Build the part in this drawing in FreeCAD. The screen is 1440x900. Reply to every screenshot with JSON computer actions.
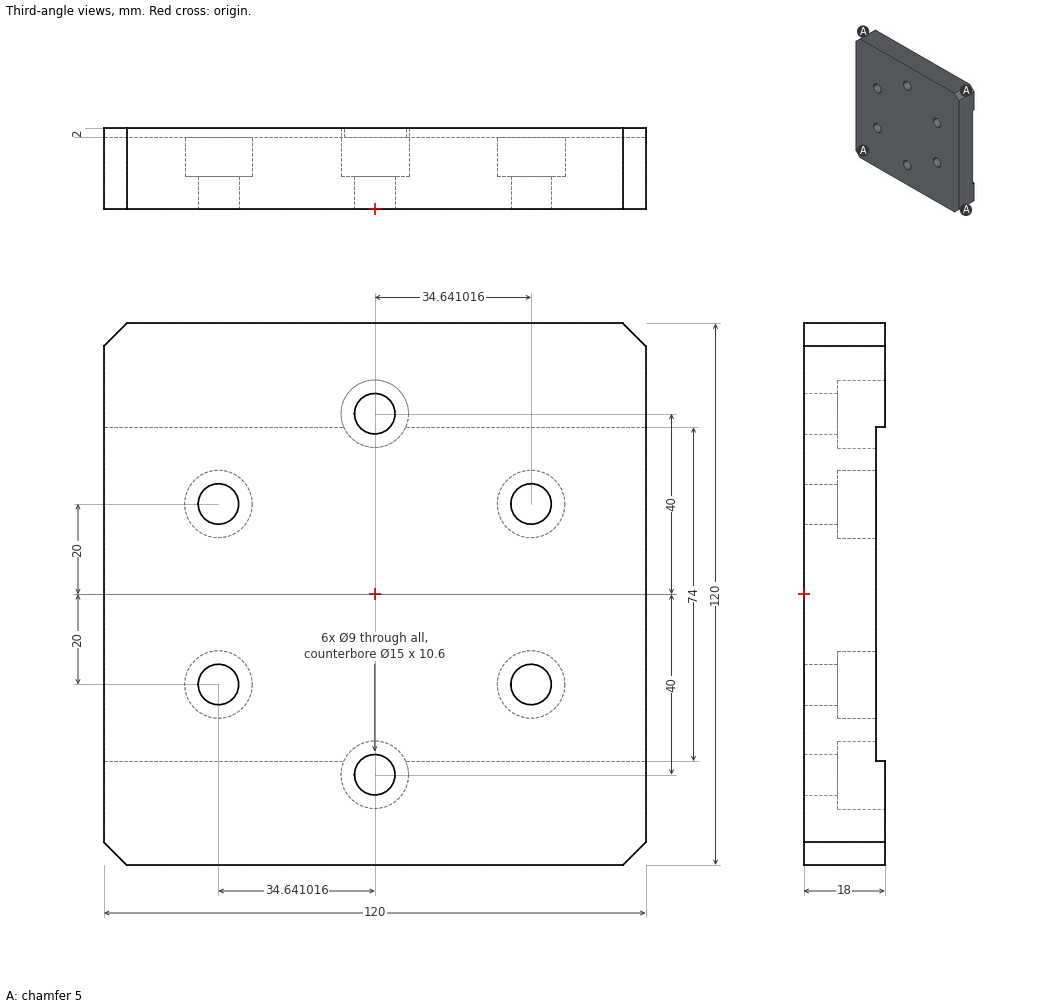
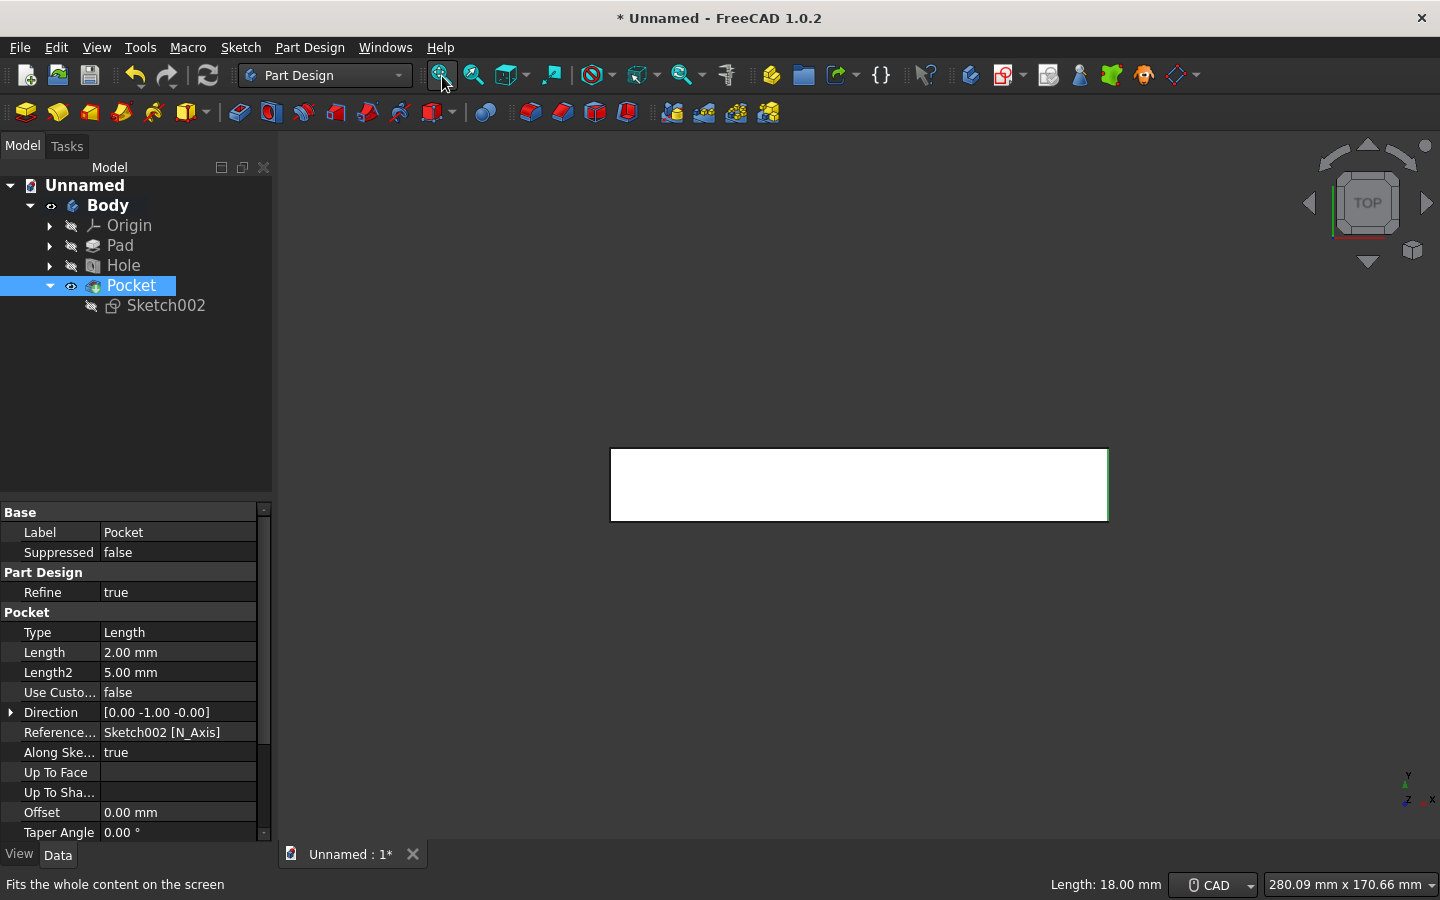
{"action": "left_click", "coordinate": [610, 484], "text": "ctrl"}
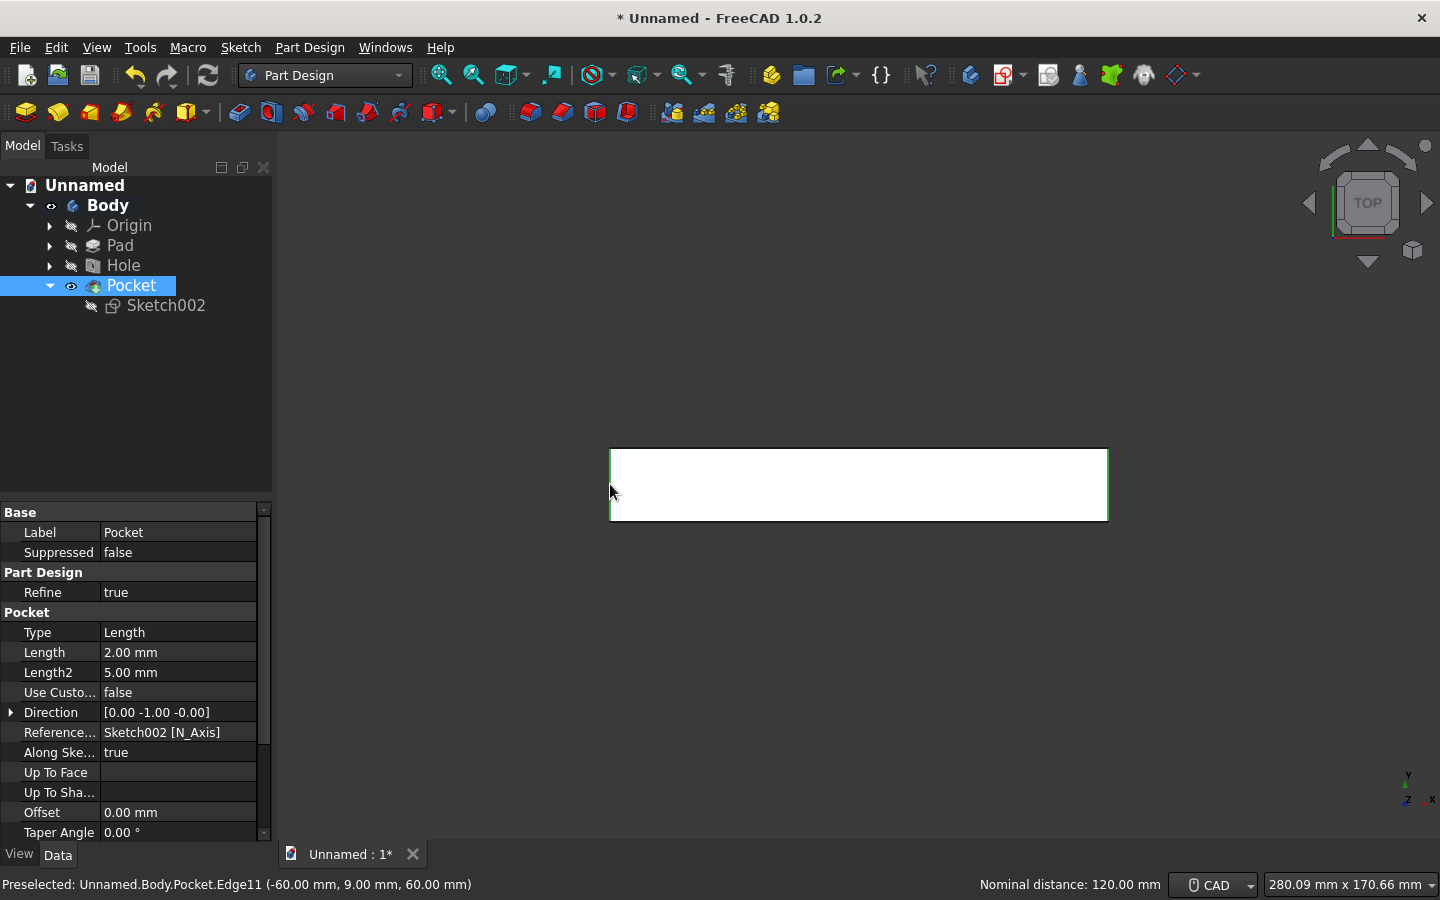
{"action": "key", "text": "1"}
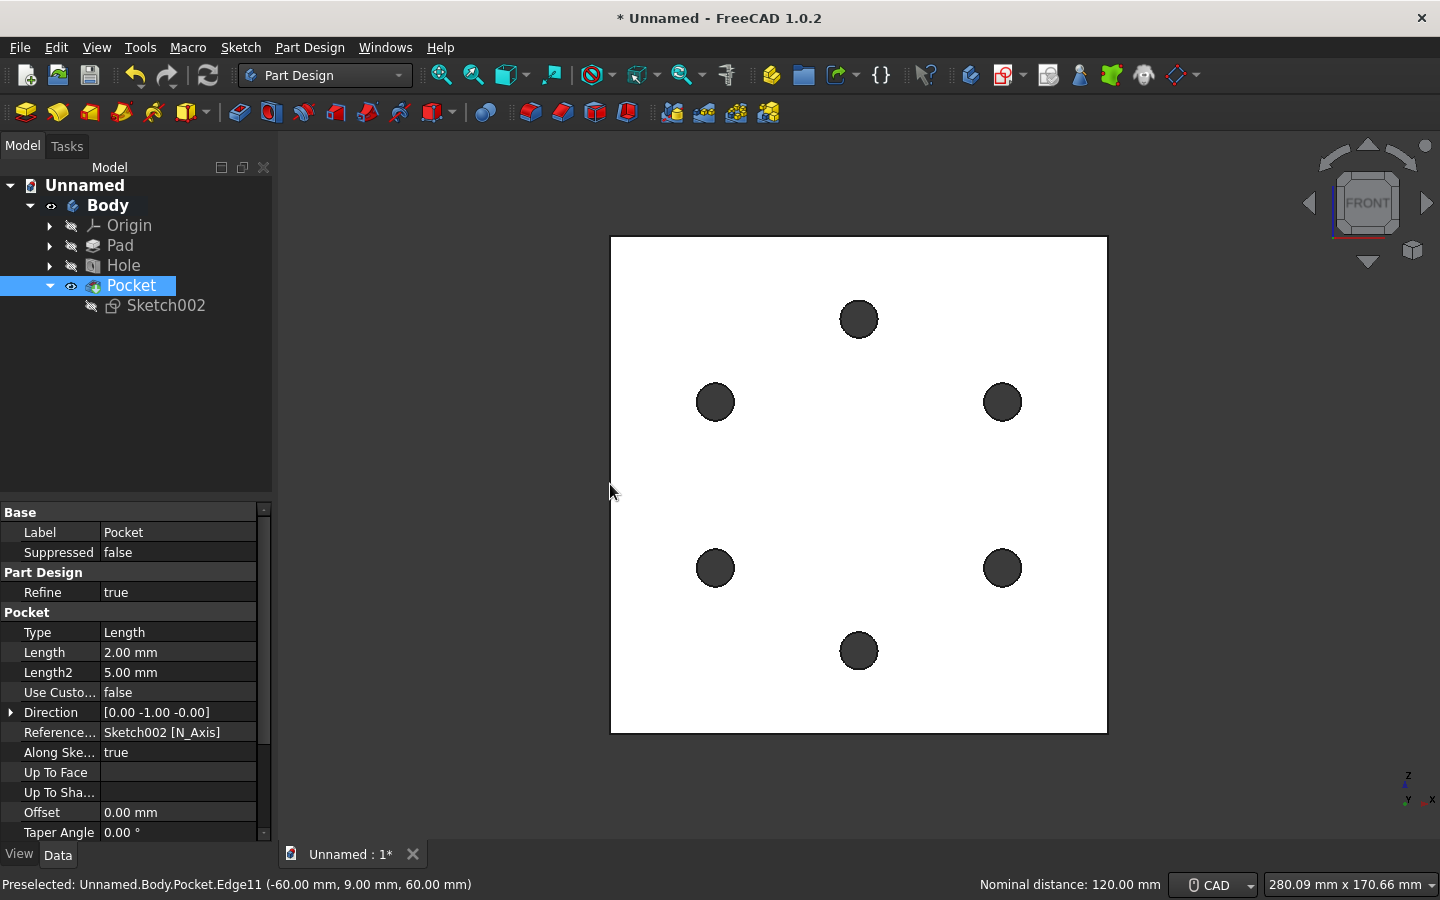
{"action": "key", "text": "3"}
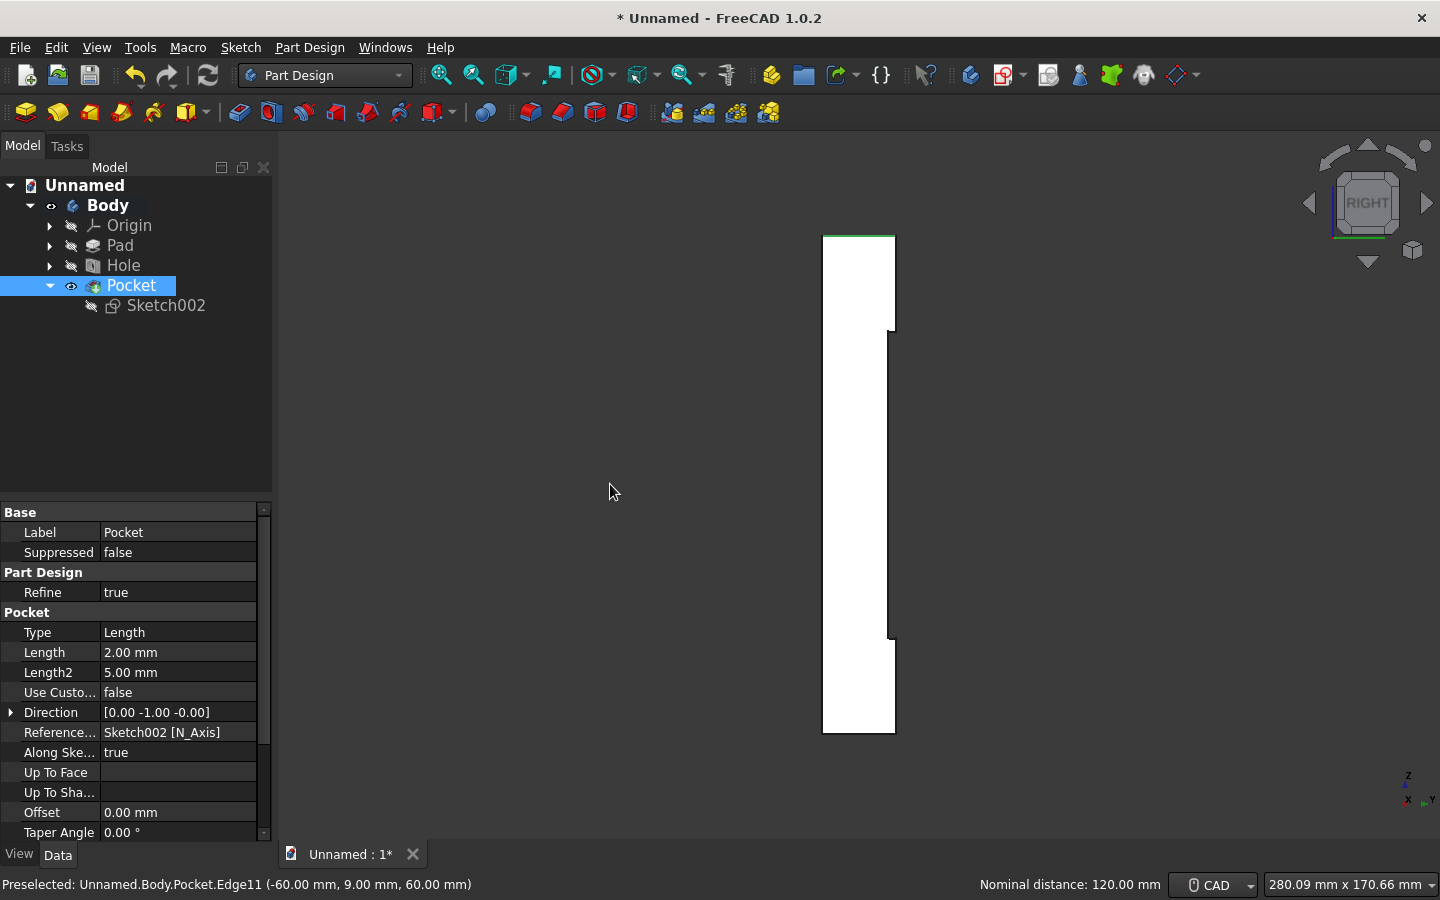
{"action": "left_click", "coordinate": [859, 733], "text": "ctrl"}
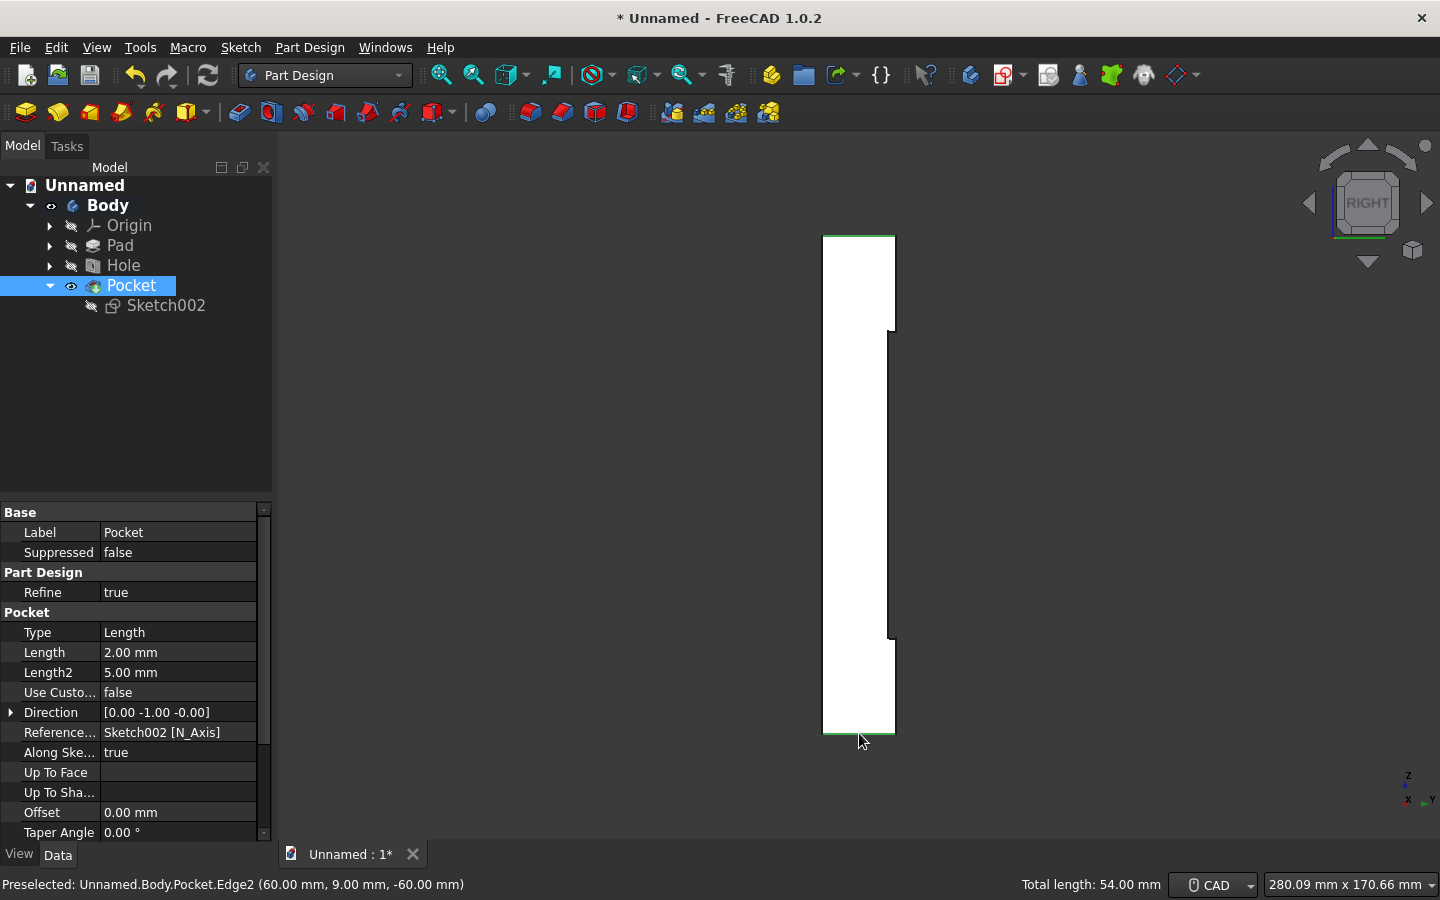
{"action": "key", "text": "5"}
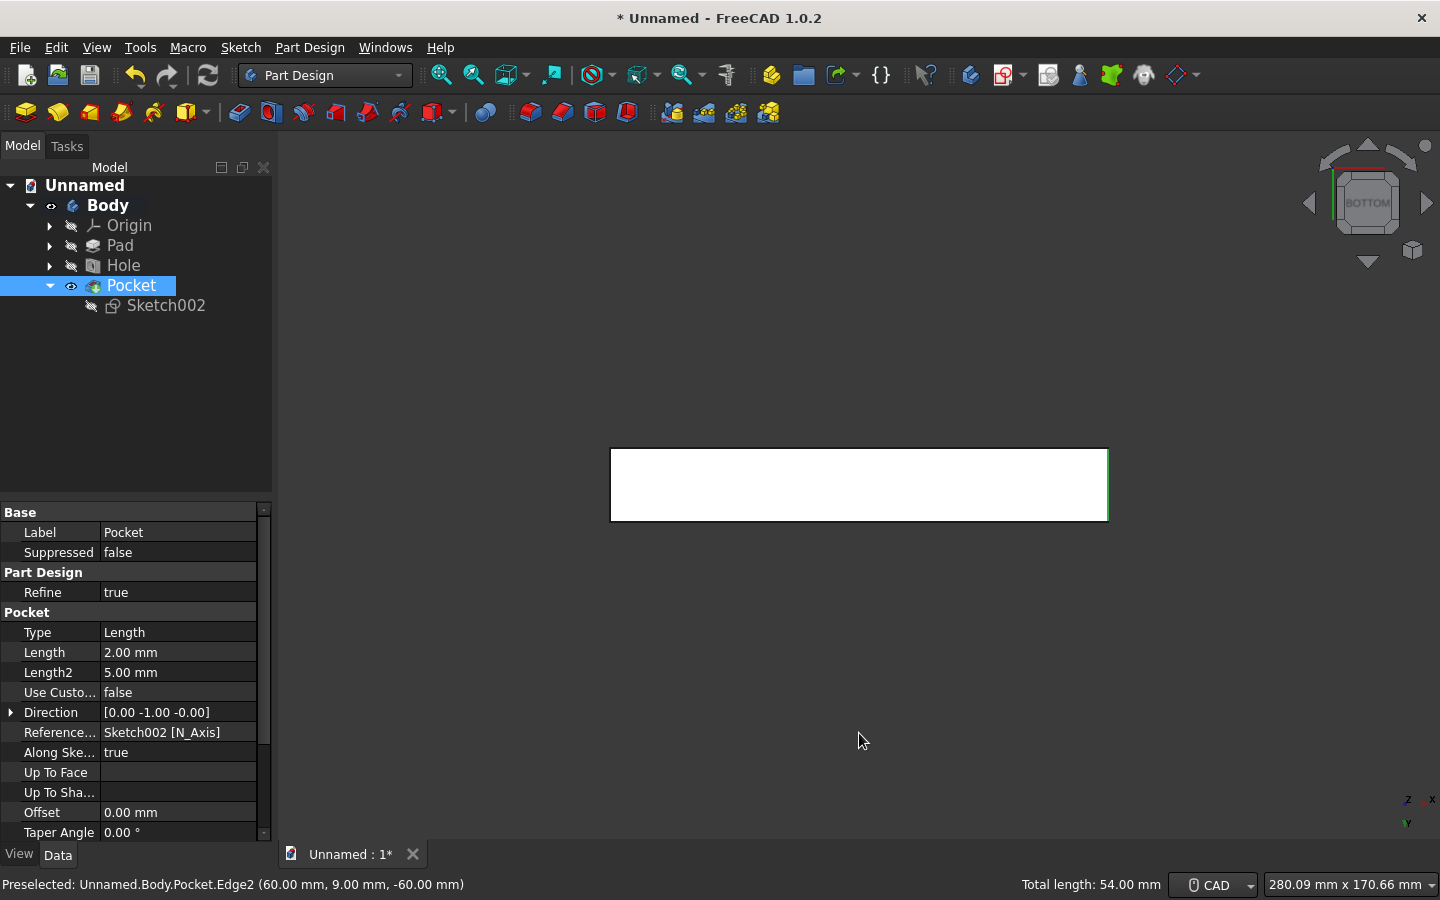
{"action": "left_click", "coordinate": [442, 76]}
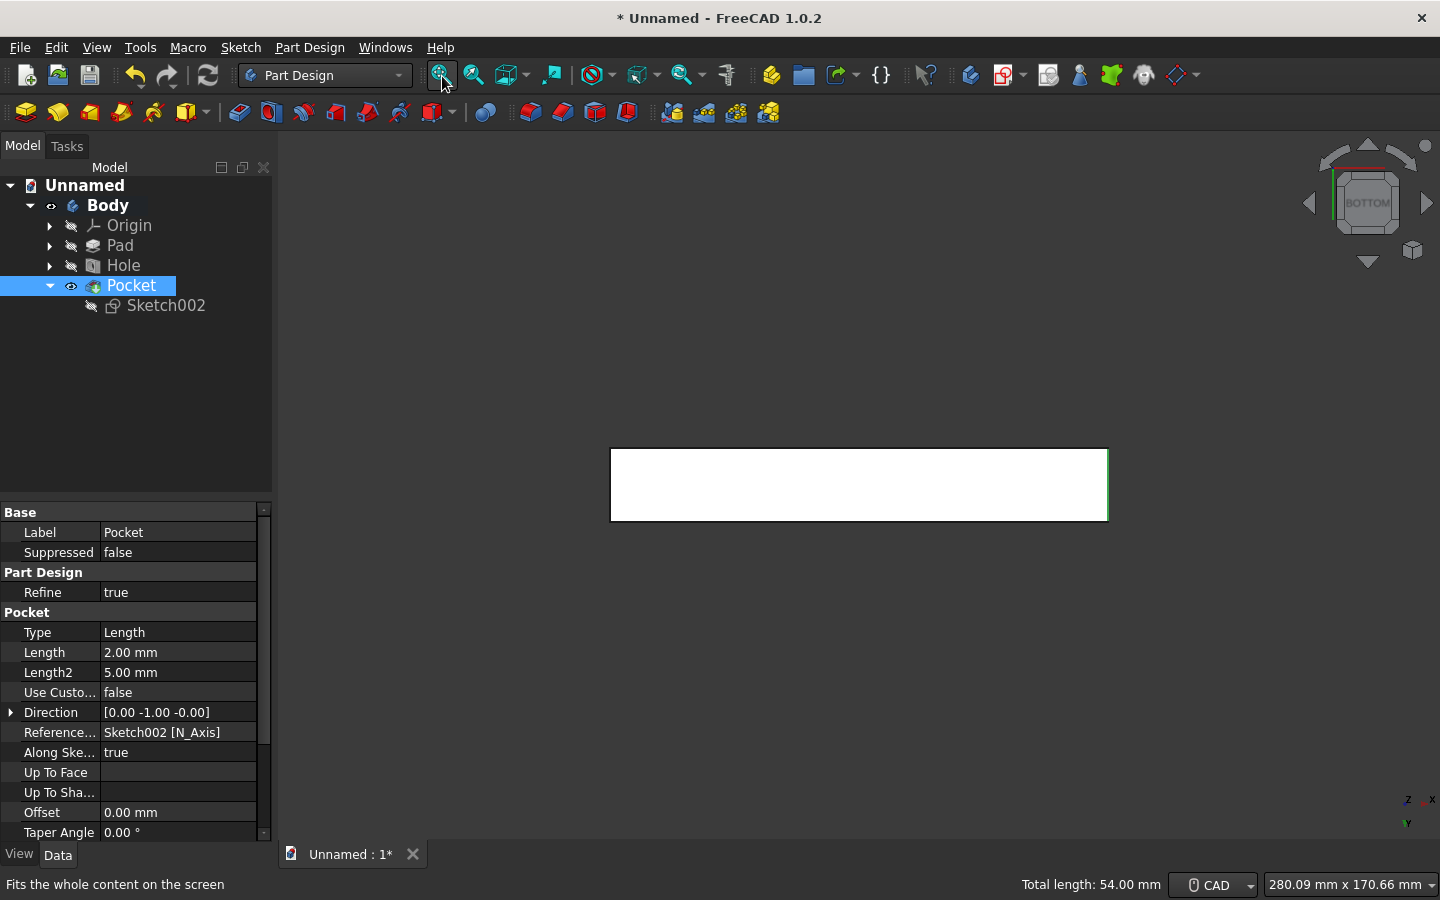
{"action": "left_click", "coordinate": [610, 484], "text": "ctrl"}